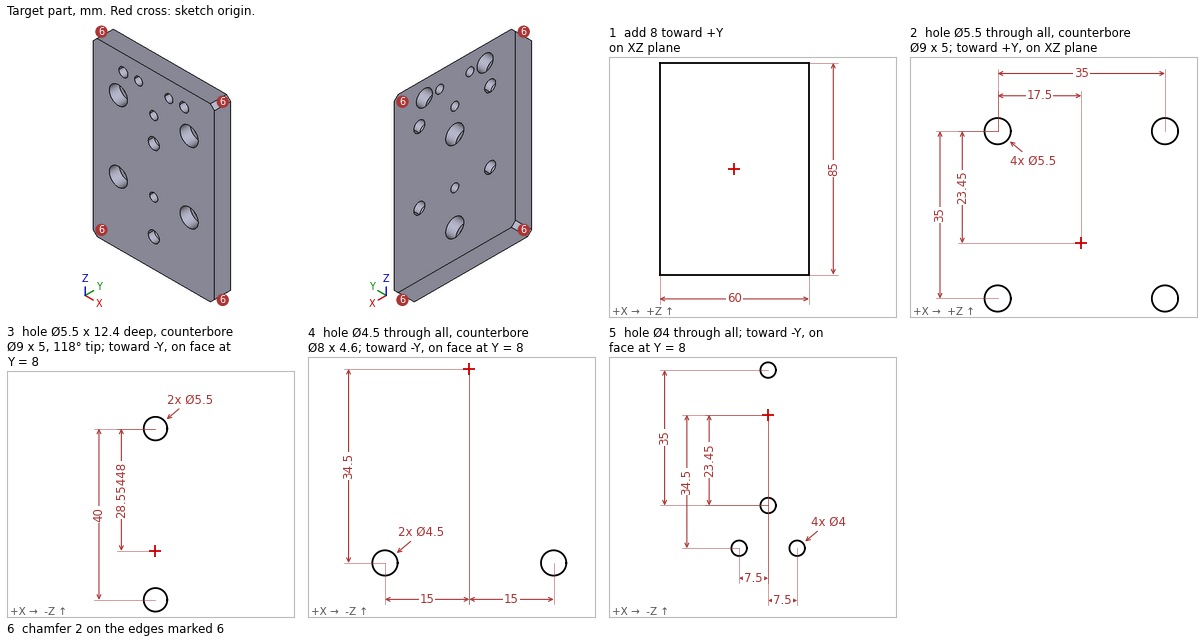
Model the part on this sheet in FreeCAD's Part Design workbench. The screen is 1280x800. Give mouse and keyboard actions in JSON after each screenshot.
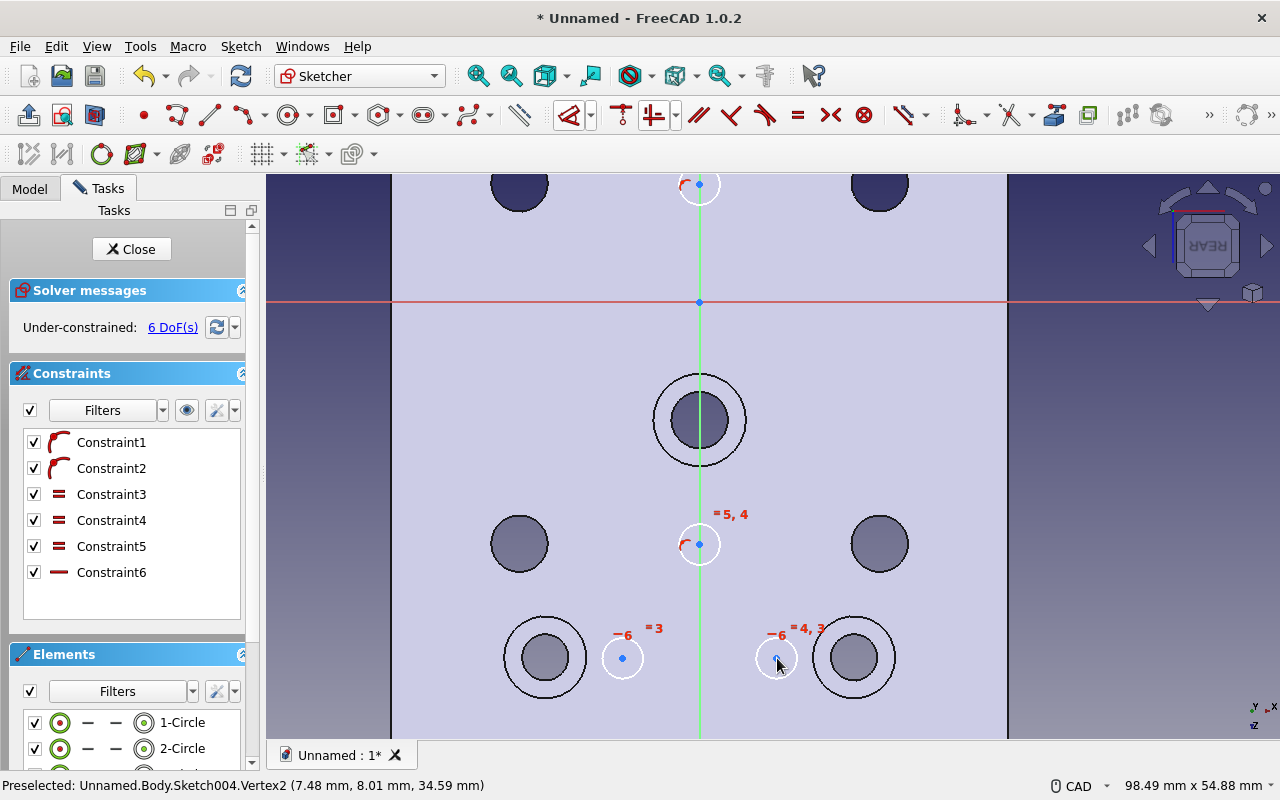
{"action": "left_click", "coordinate": [637, 644]}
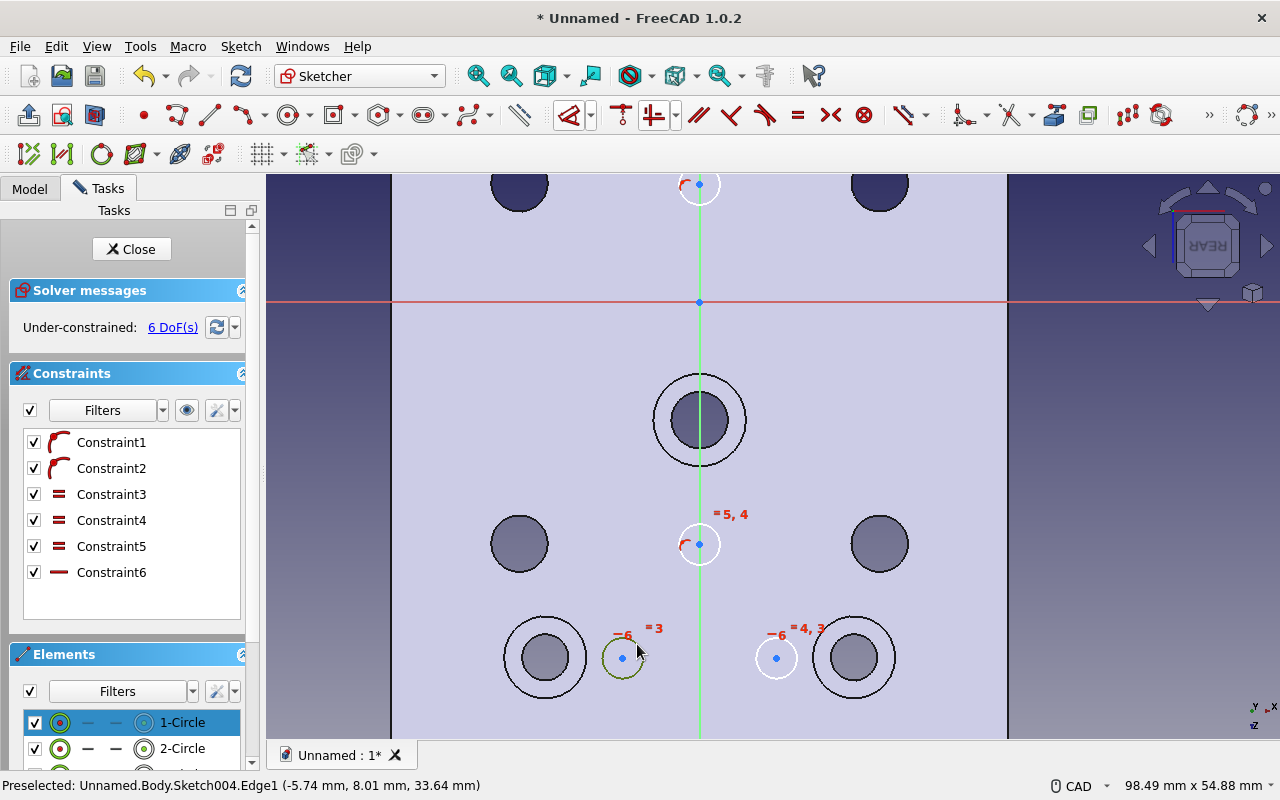
{"action": "key", "text": "k o"}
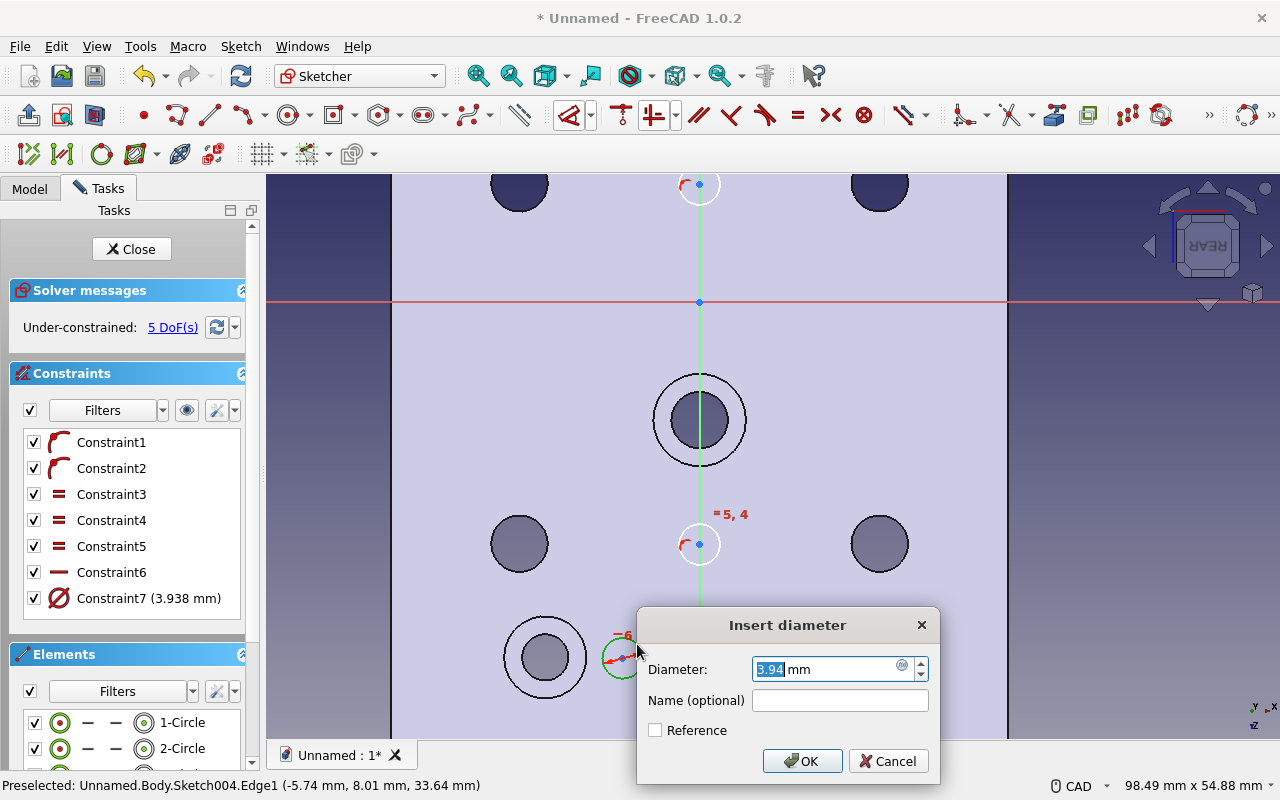
{"action": "type", "text": "4"}
{"action": "key", "text": "Return"}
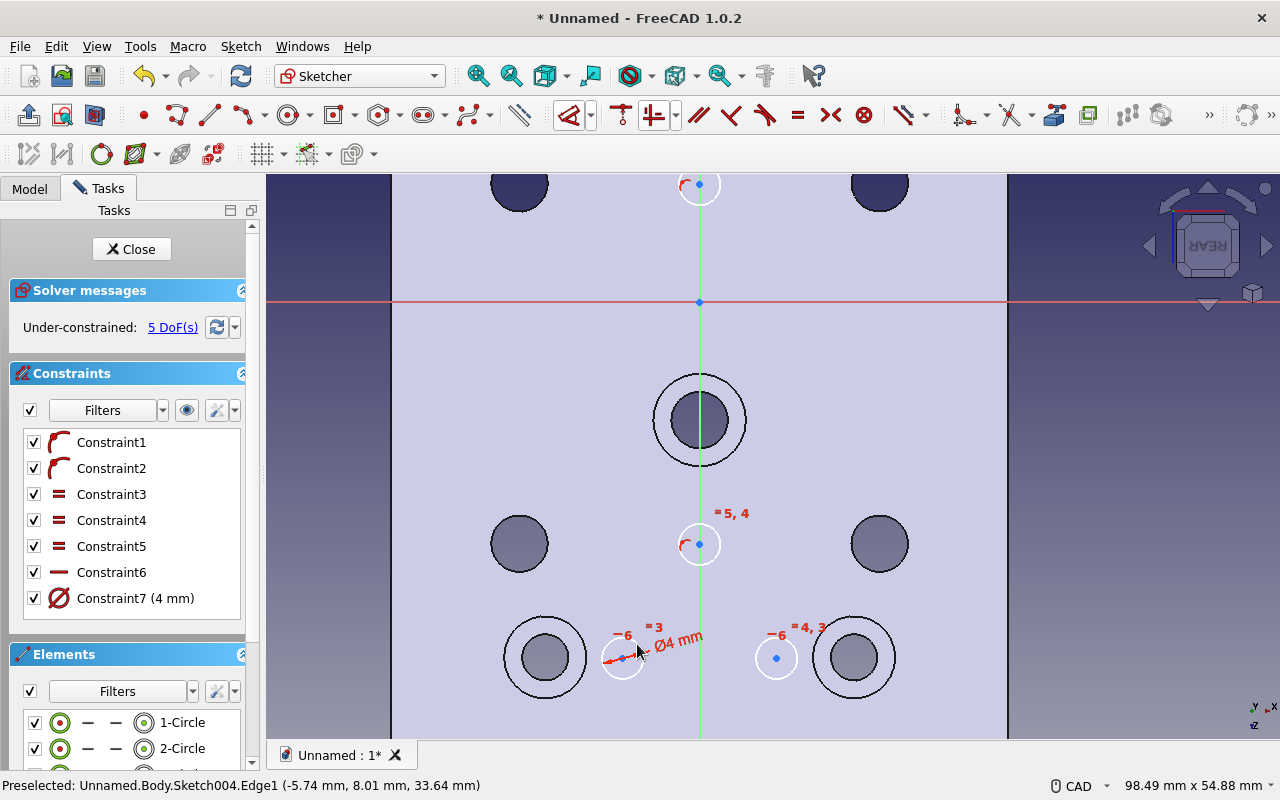
{"action": "left_click", "coordinate": [623, 658]}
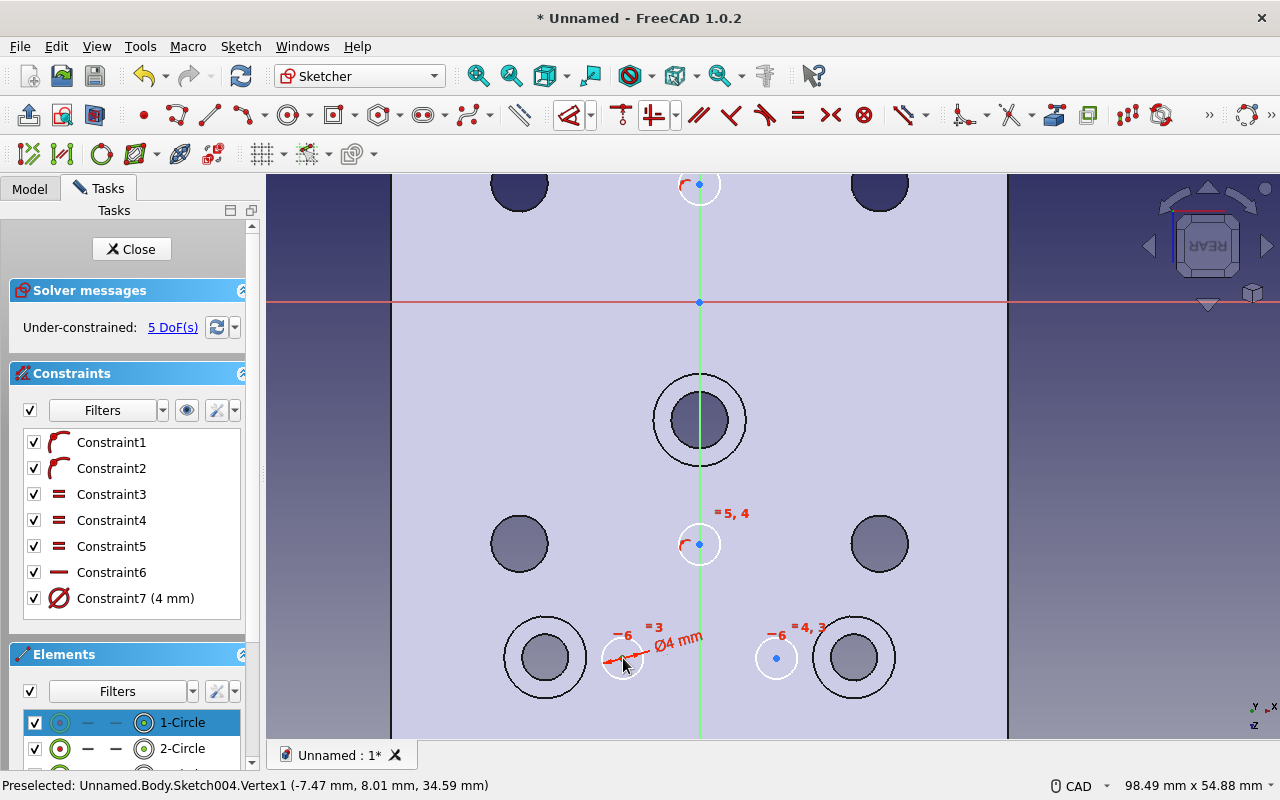
{"action": "left_click", "coordinate": [590, 116]}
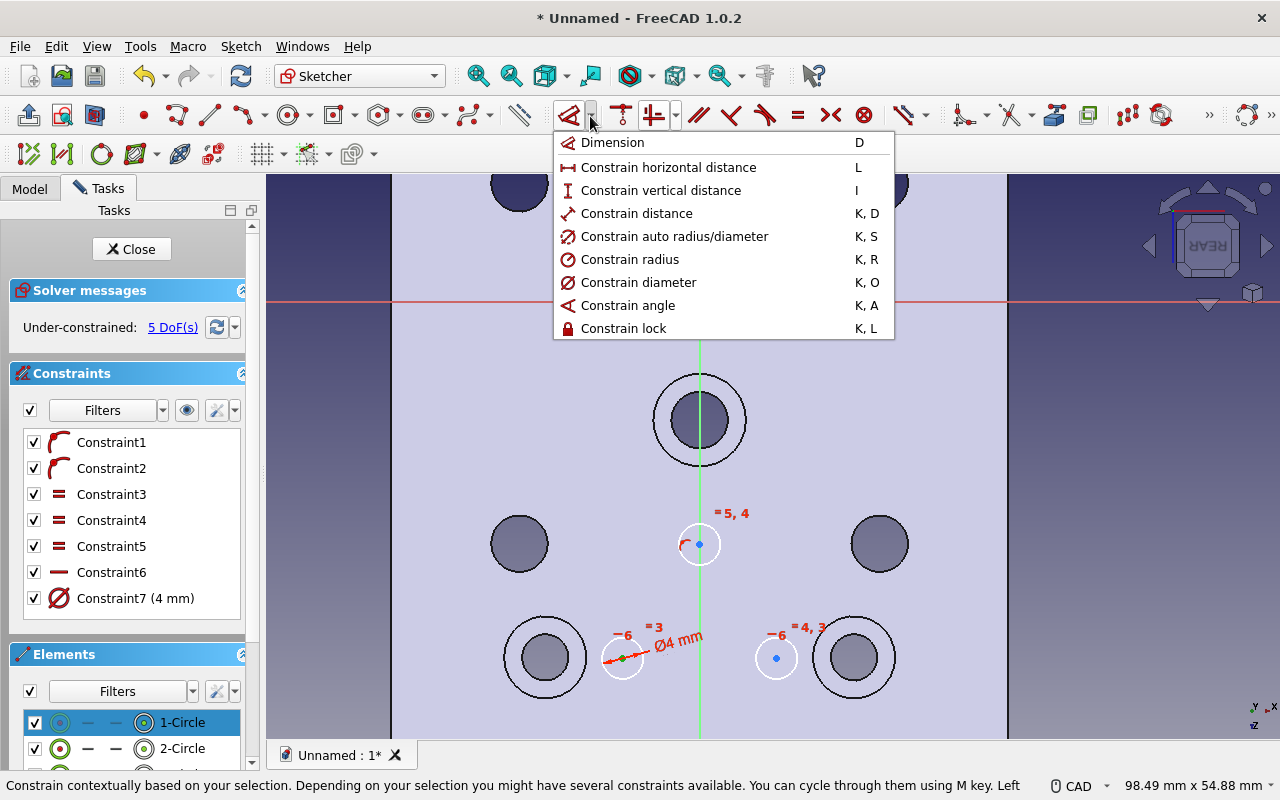
{"action": "left_click", "coordinate": [724, 168]}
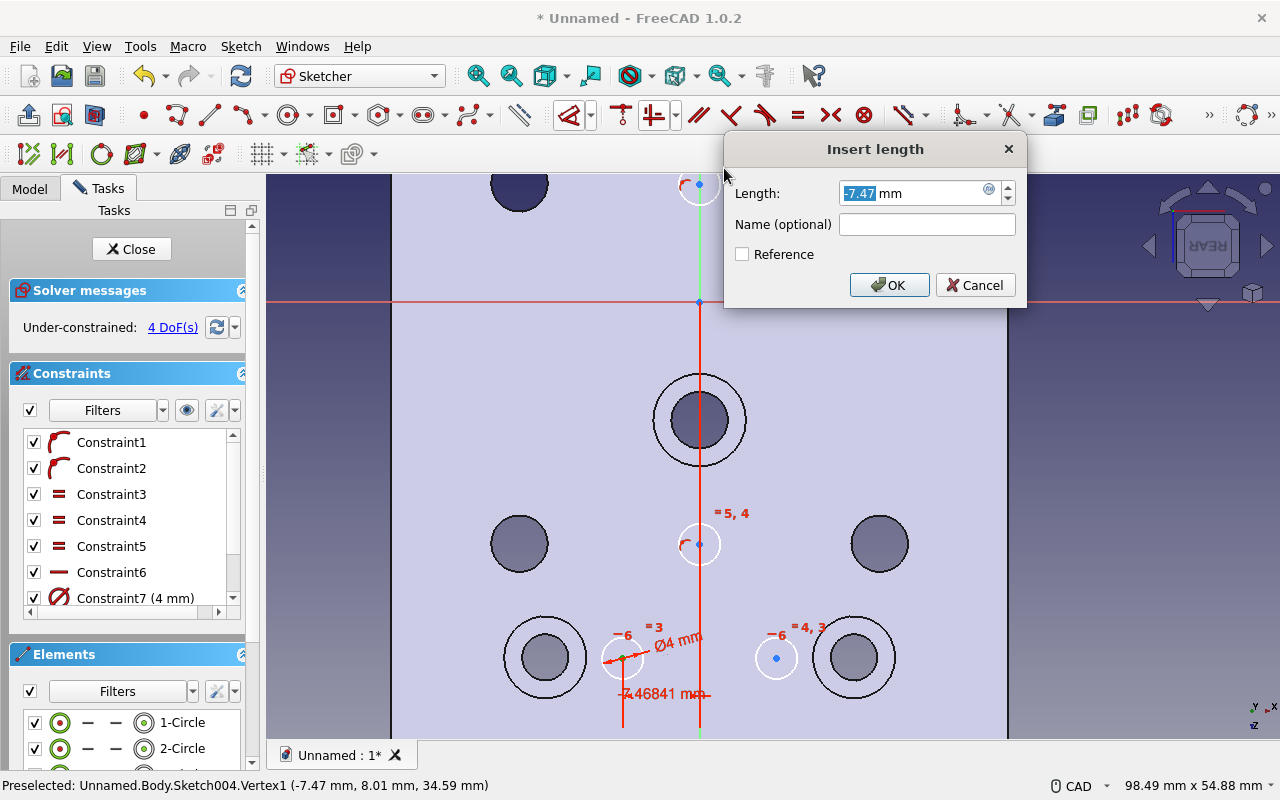
{"action": "type", "text": "-7.5"}
{"action": "key", "text": "Return"}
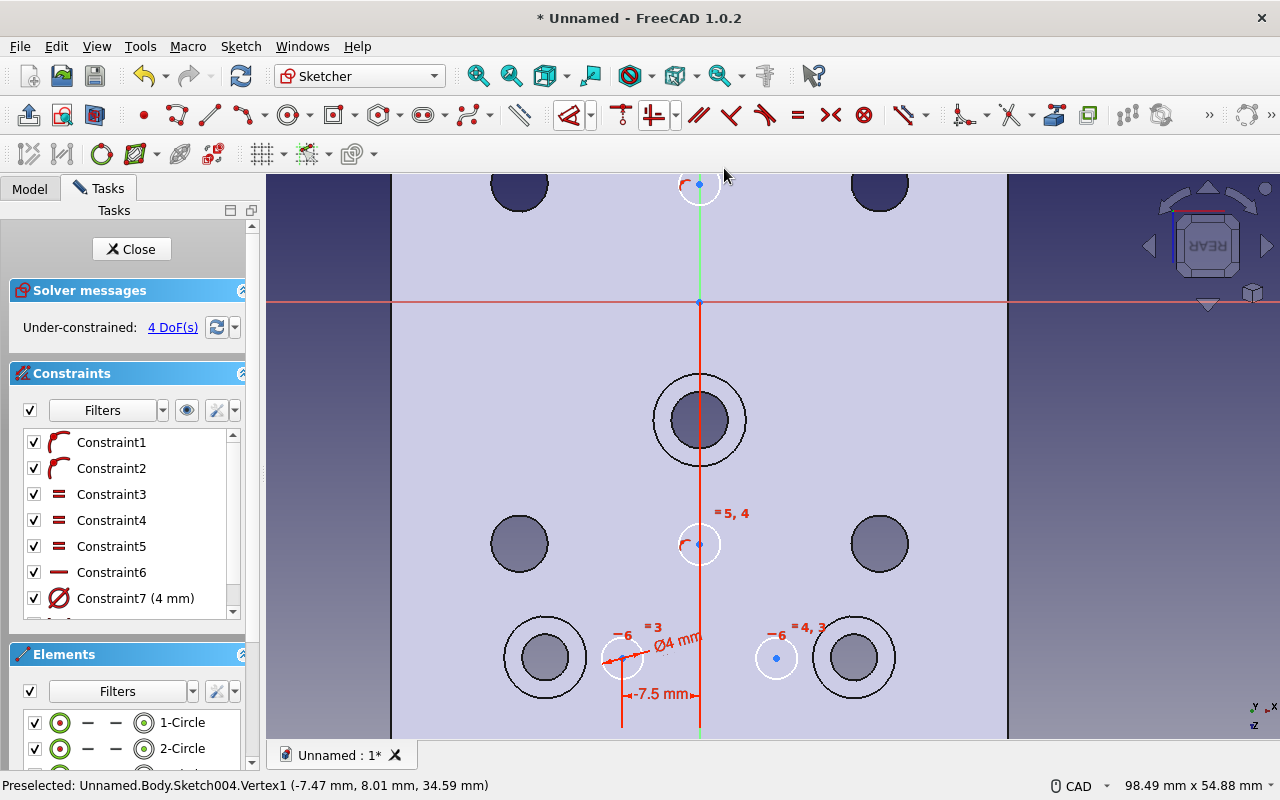
{"action": "left_click", "coordinate": [777, 658]}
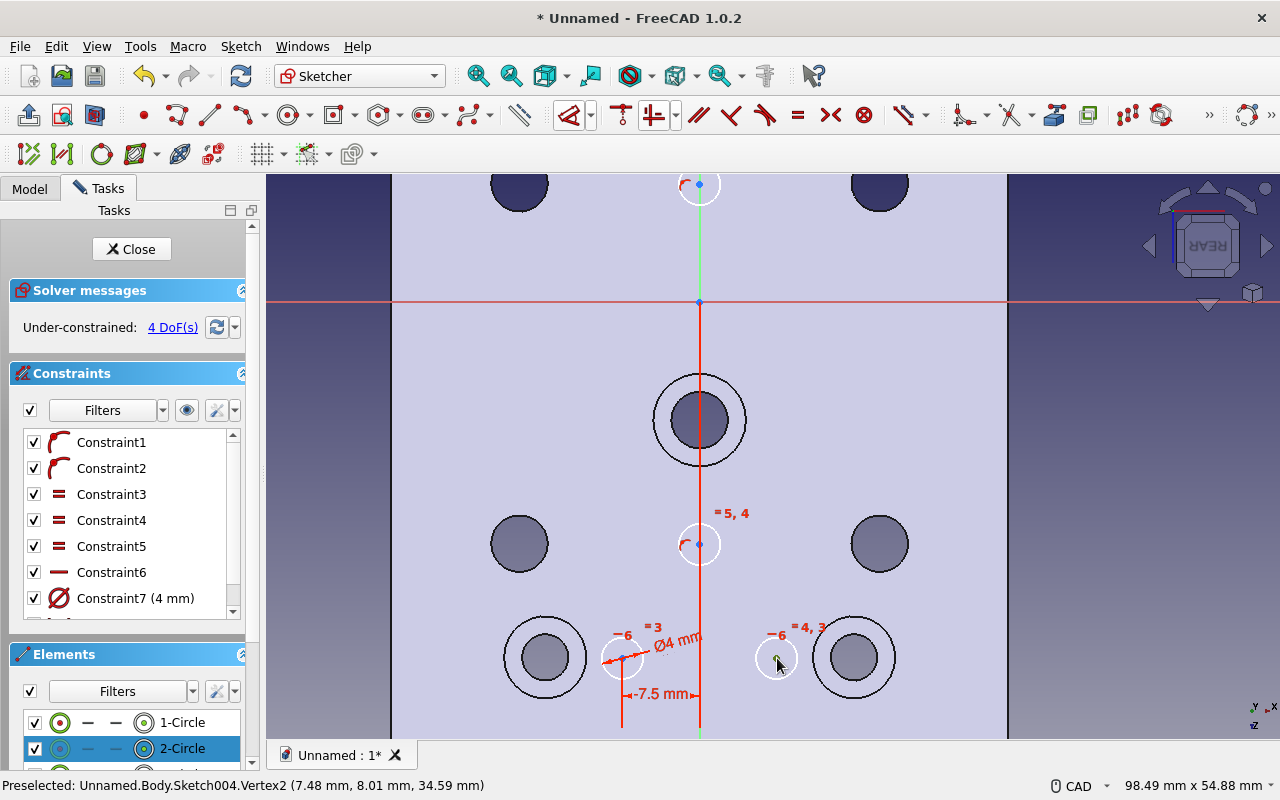
{"action": "key", "text": "l"}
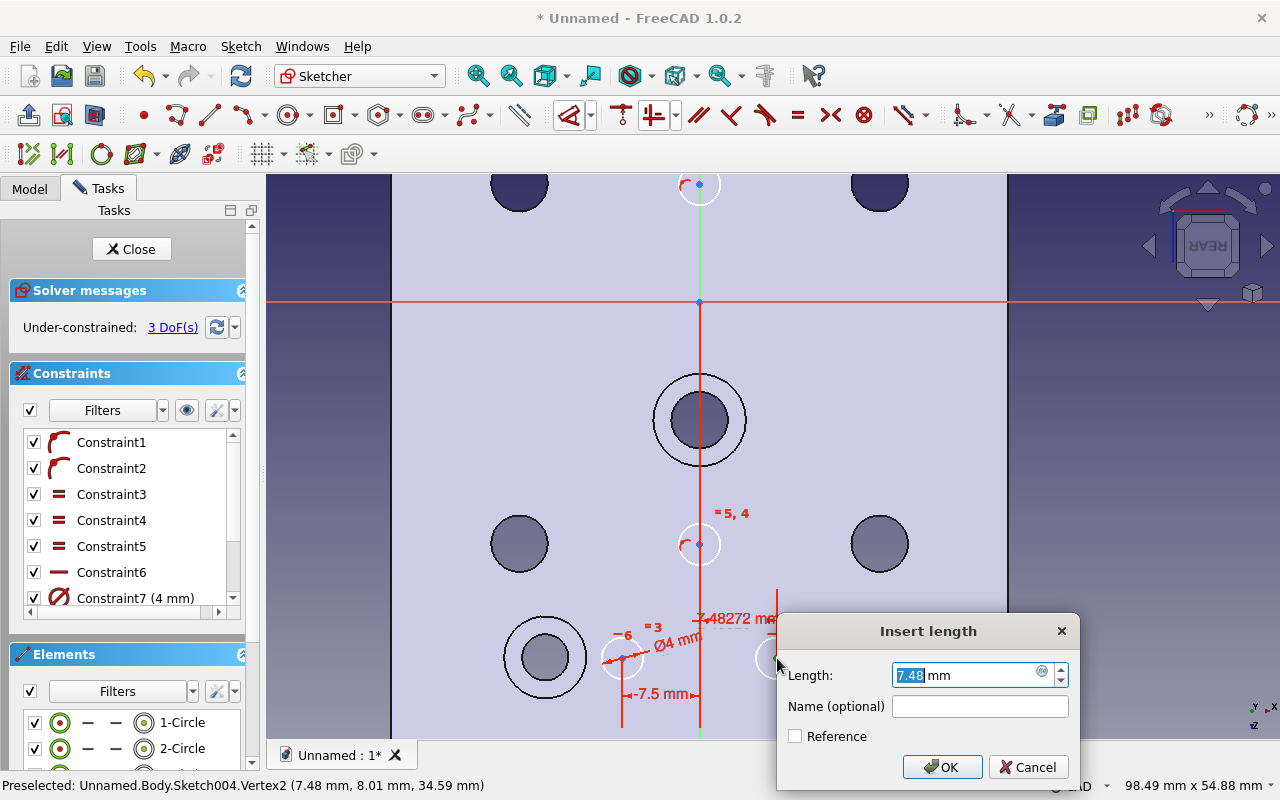
{"action": "type", "text": "7.5"}
{"action": "key", "text": "Return"}